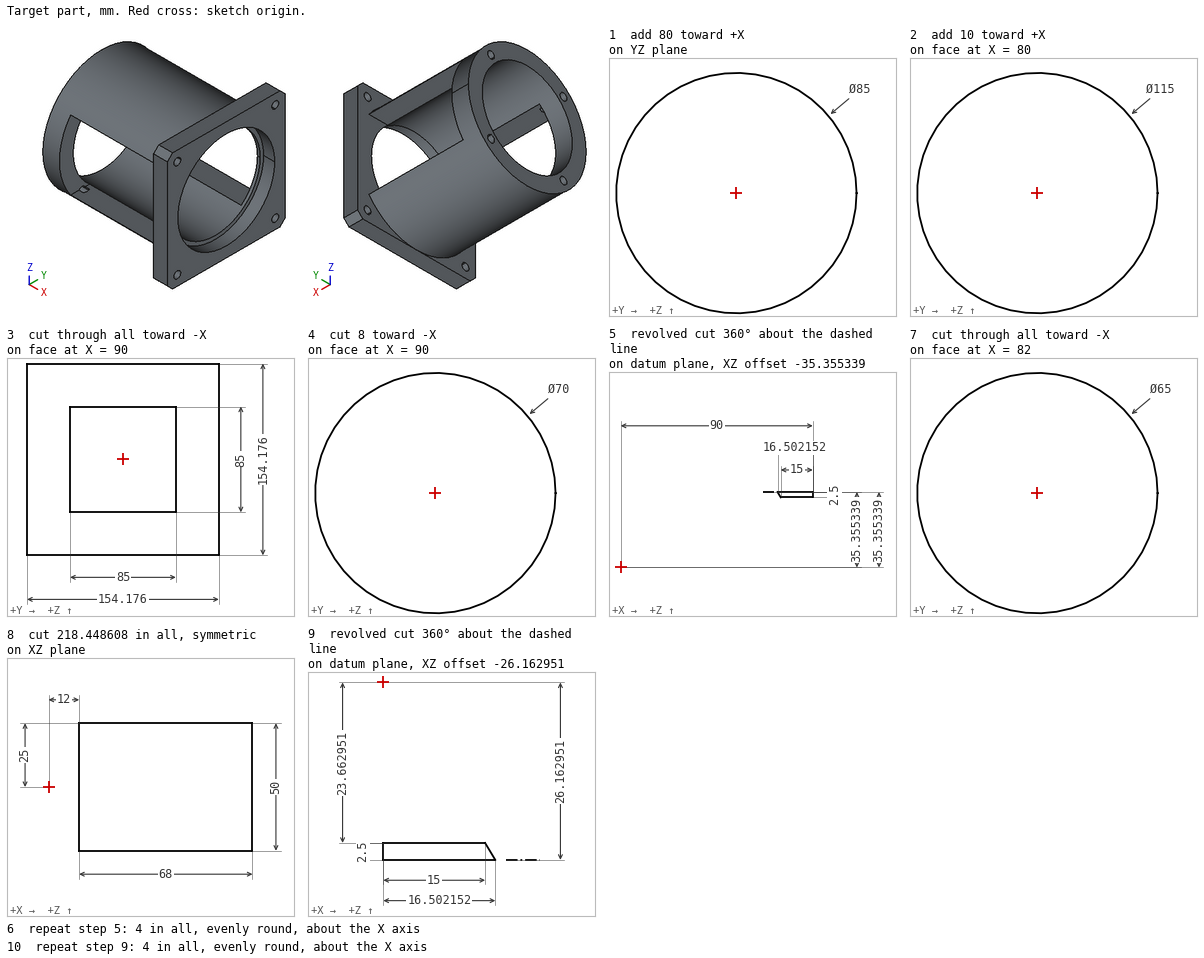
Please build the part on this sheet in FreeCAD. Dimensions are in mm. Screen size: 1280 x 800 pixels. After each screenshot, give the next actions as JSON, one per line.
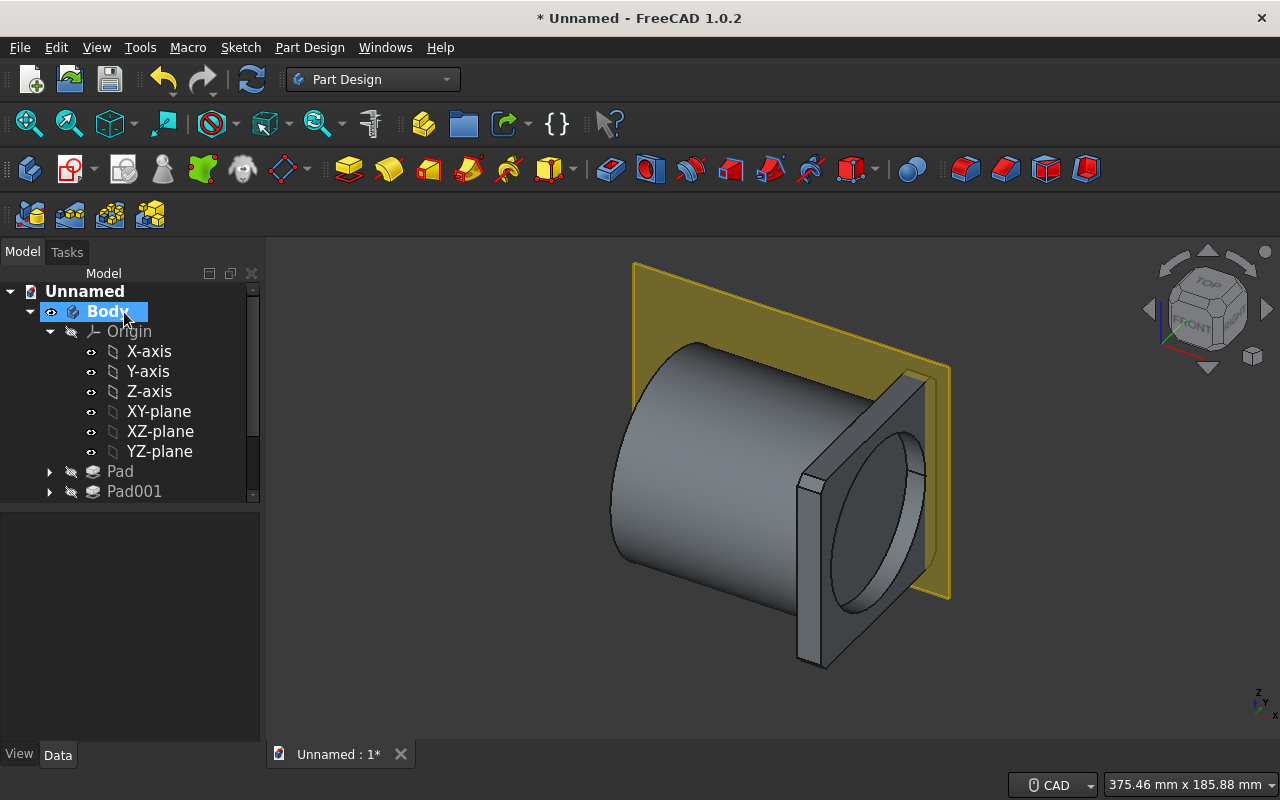
{"action": "scroll", "coordinate": [100, 387], "scroll_direction": "down", "scroll_amount": 3}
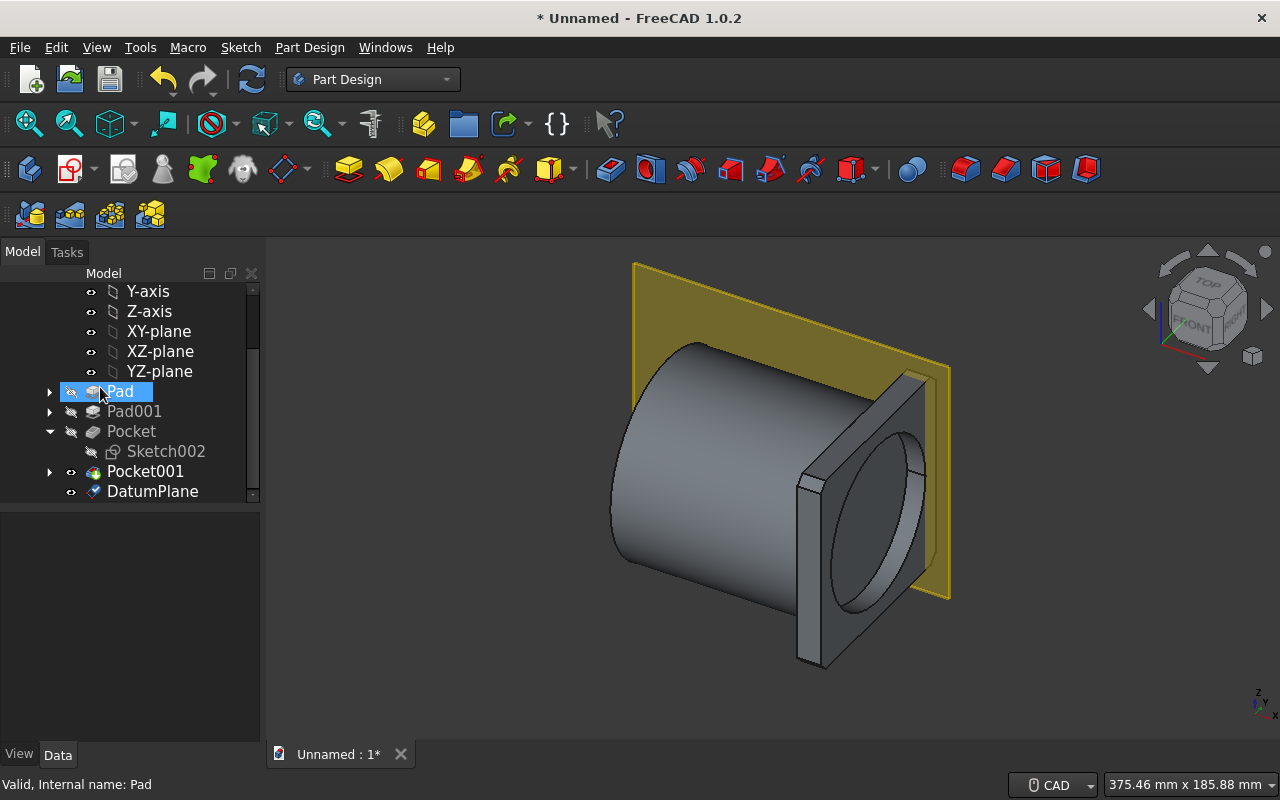
{"action": "left_click", "coordinate": [116, 492]}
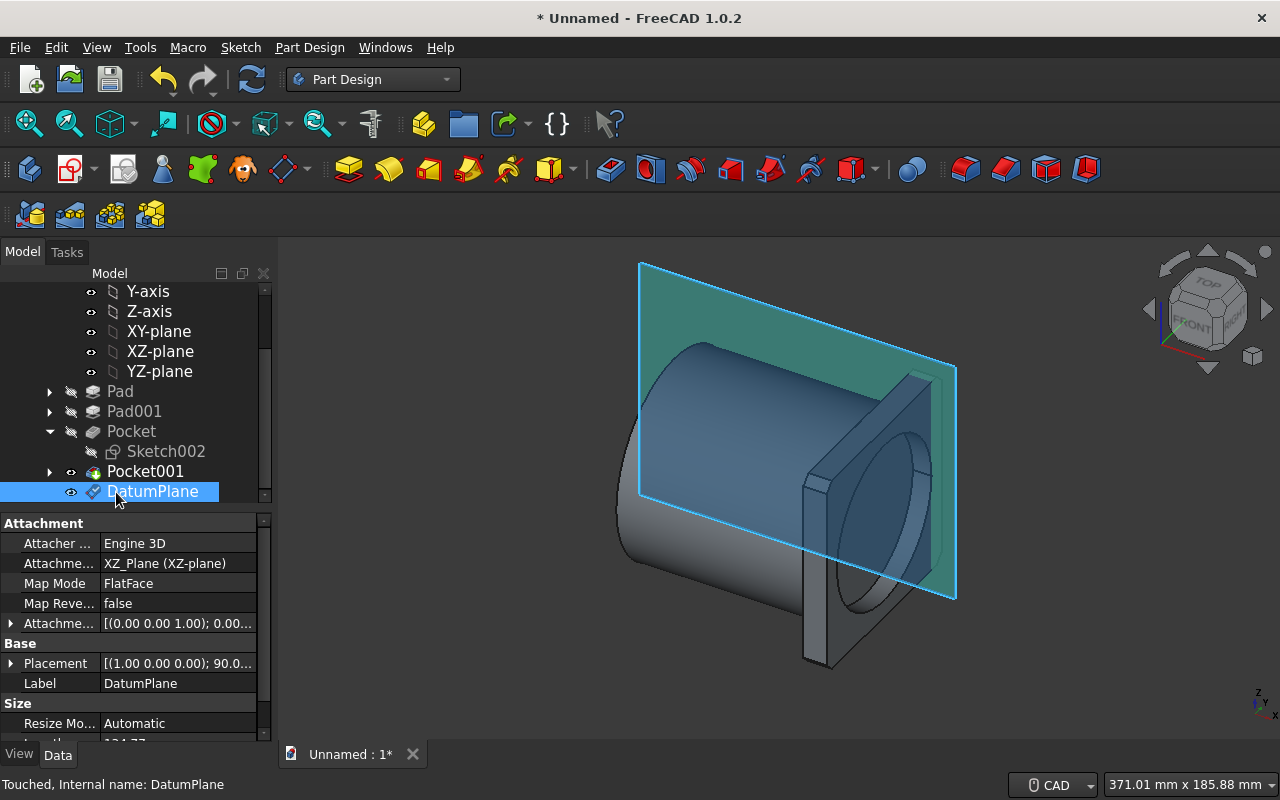
{"action": "left_click", "coordinate": [70, 170]}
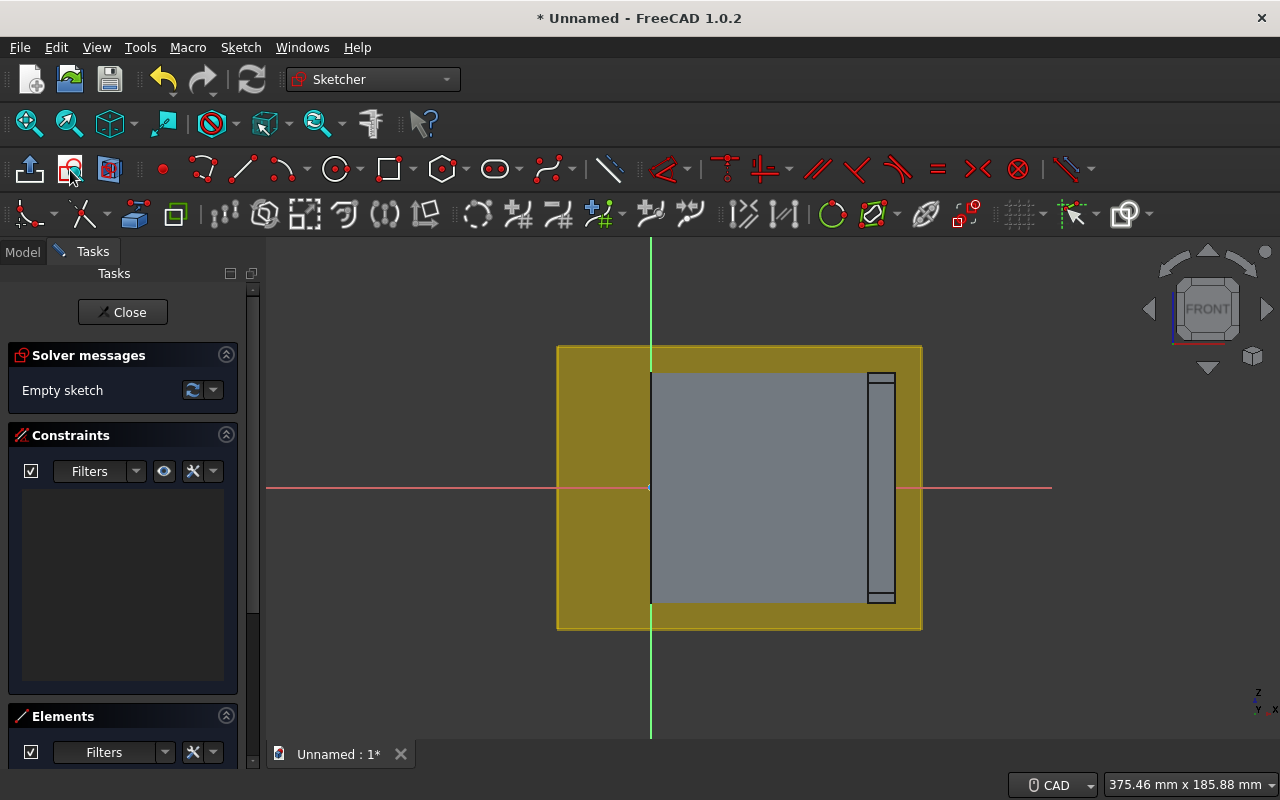
{"action": "left_click", "coordinate": [110, 170]}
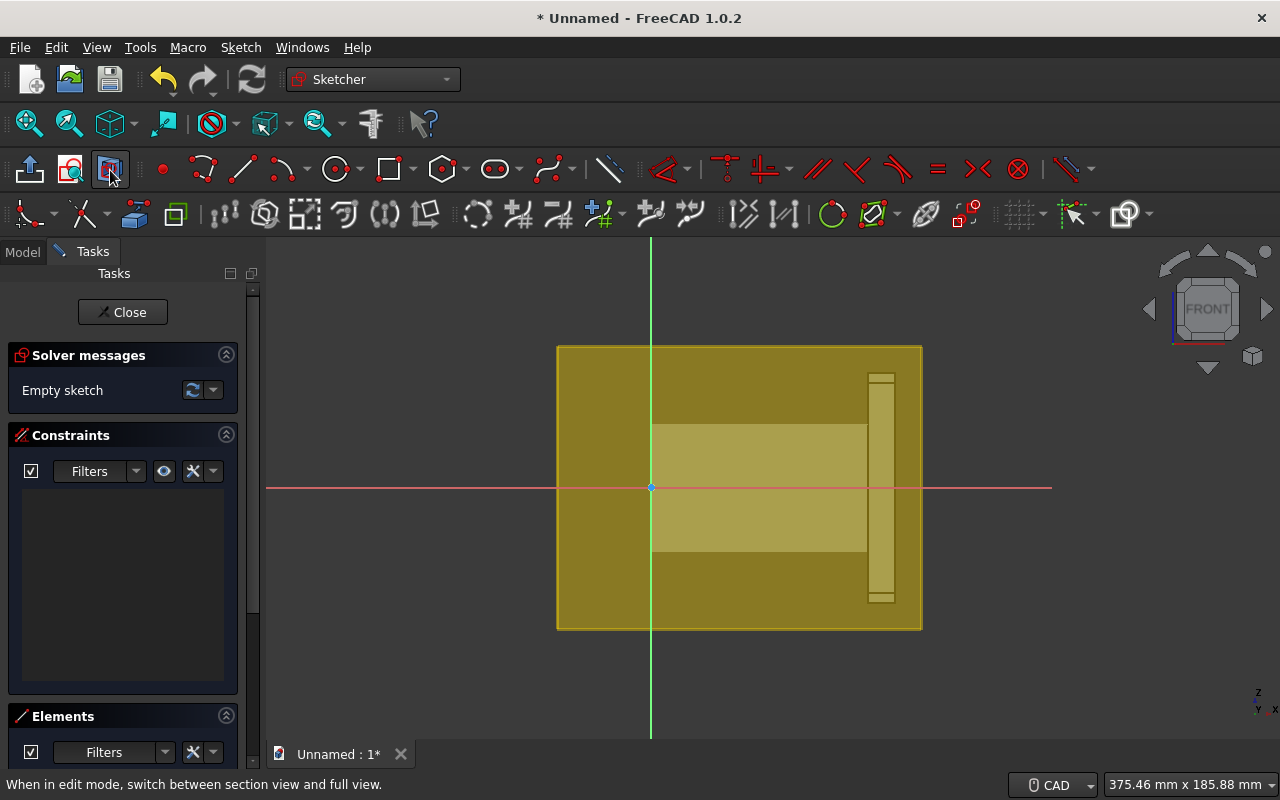
{"action": "scroll", "coordinate": [883, 384], "scroll_direction": "up", "scroll_amount": 11}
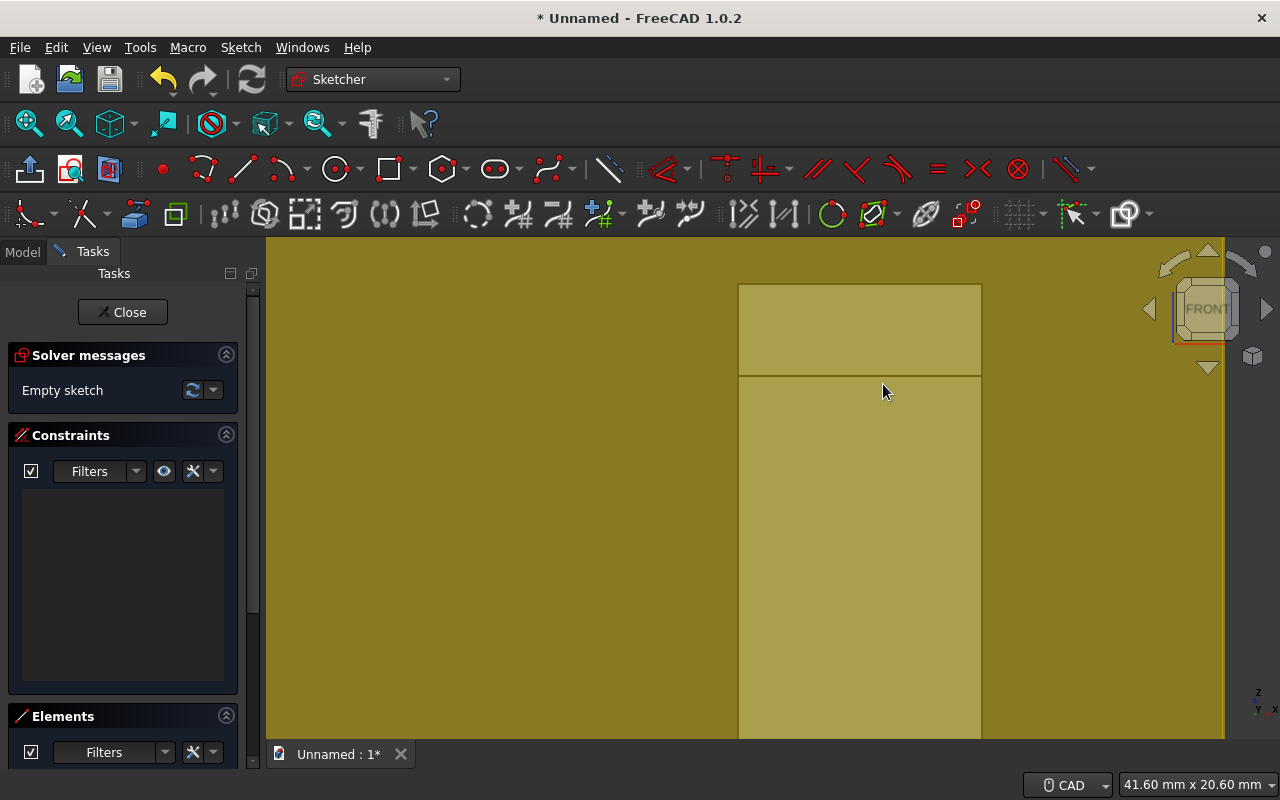
{"action": "left_click", "coordinate": [204, 170]}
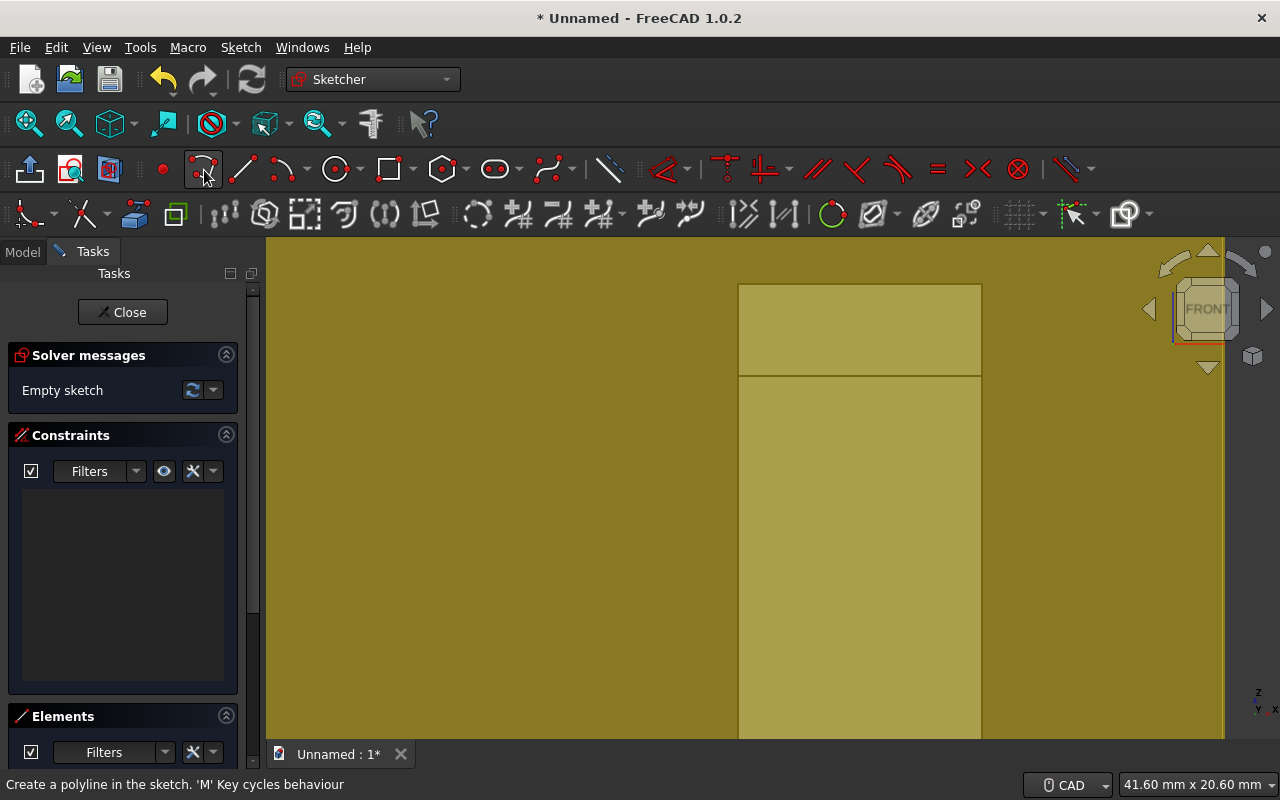
{"action": "left_click", "coordinate": [580, 458]}
{"action": "left_click", "coordinate": [982, 458]}
{"action": "left_click", "coordinate": [982, 519]}
{"action": "left_click", "coordinate": [617, 519]}
{"action": "left_click", "coordinate": [580, 459]}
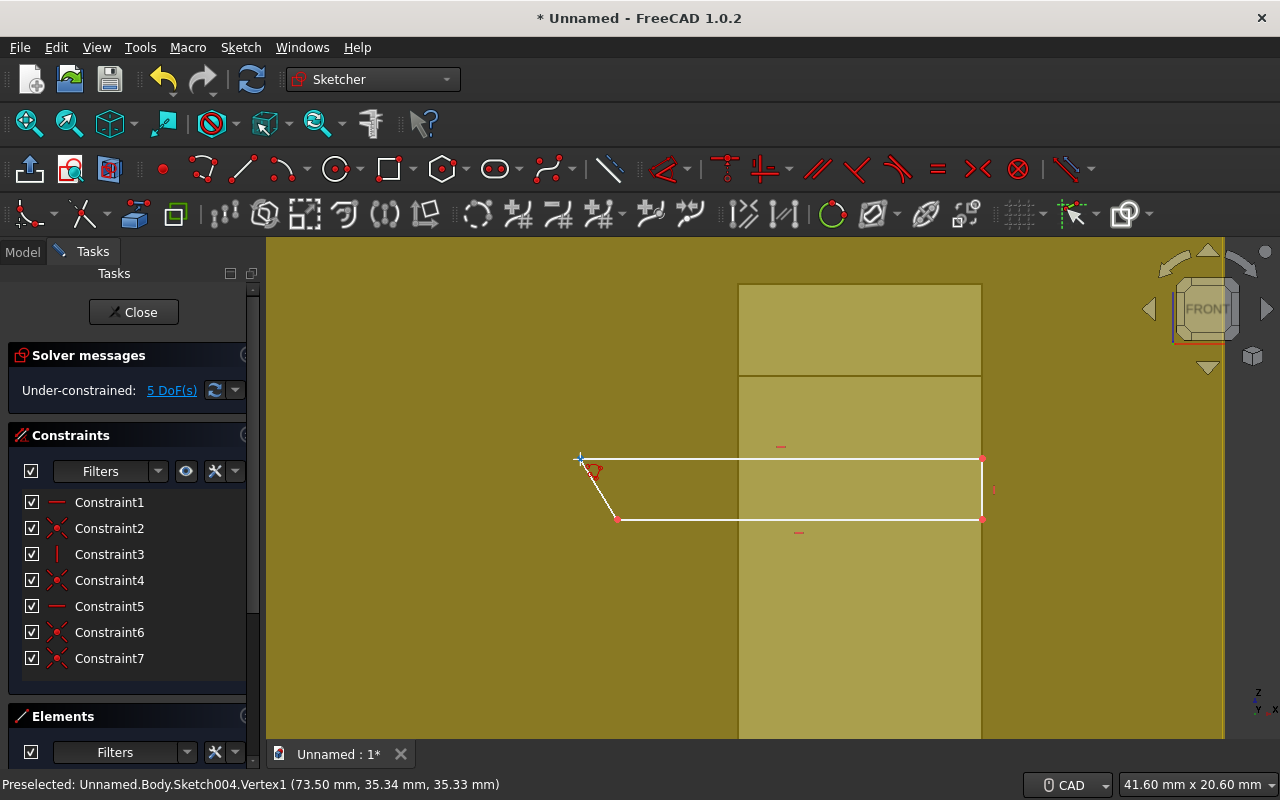
{"action": "left_click", "coordinate": [244, 170]}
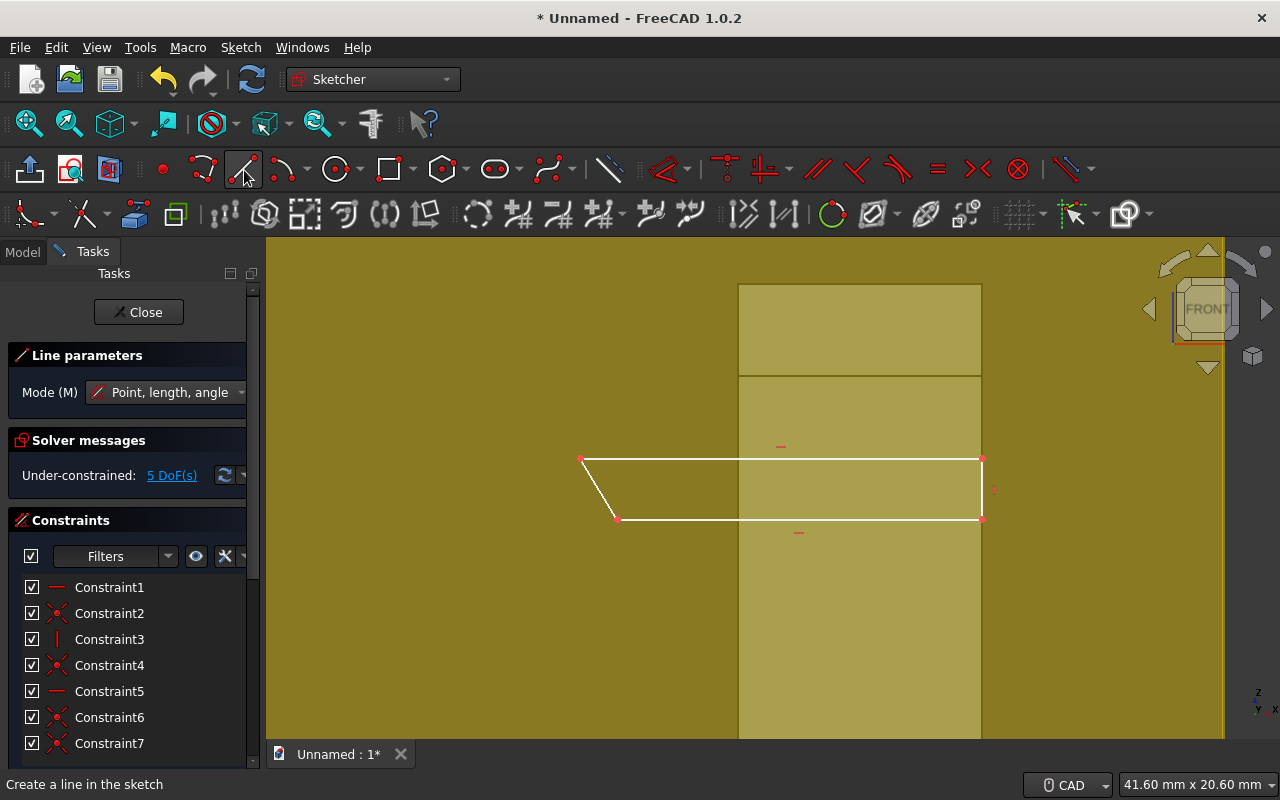
{"action": "left_click", "coordinate": [540, 458]}
{"action": "left_click", "coordinate": [419, 458]}
{"action": "key", "text": "Escape"}